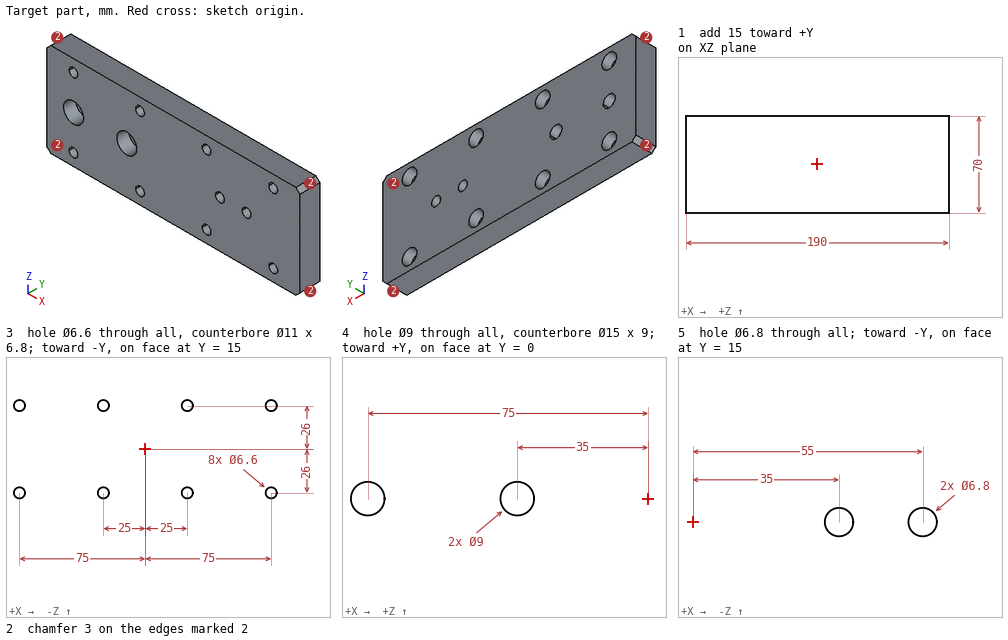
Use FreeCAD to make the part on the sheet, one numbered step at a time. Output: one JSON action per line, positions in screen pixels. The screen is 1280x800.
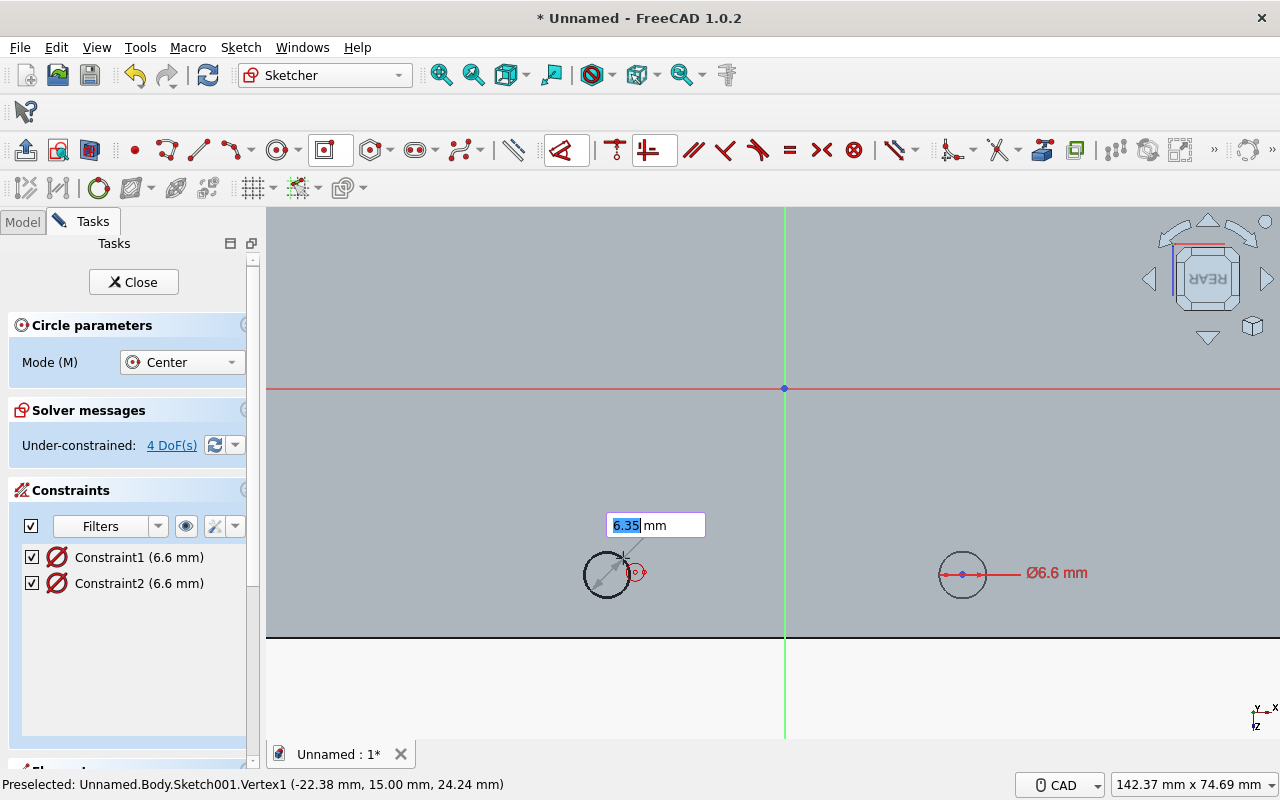
{"action": "type", "text": "6.6"}
{"action": "key", "text": "Return"}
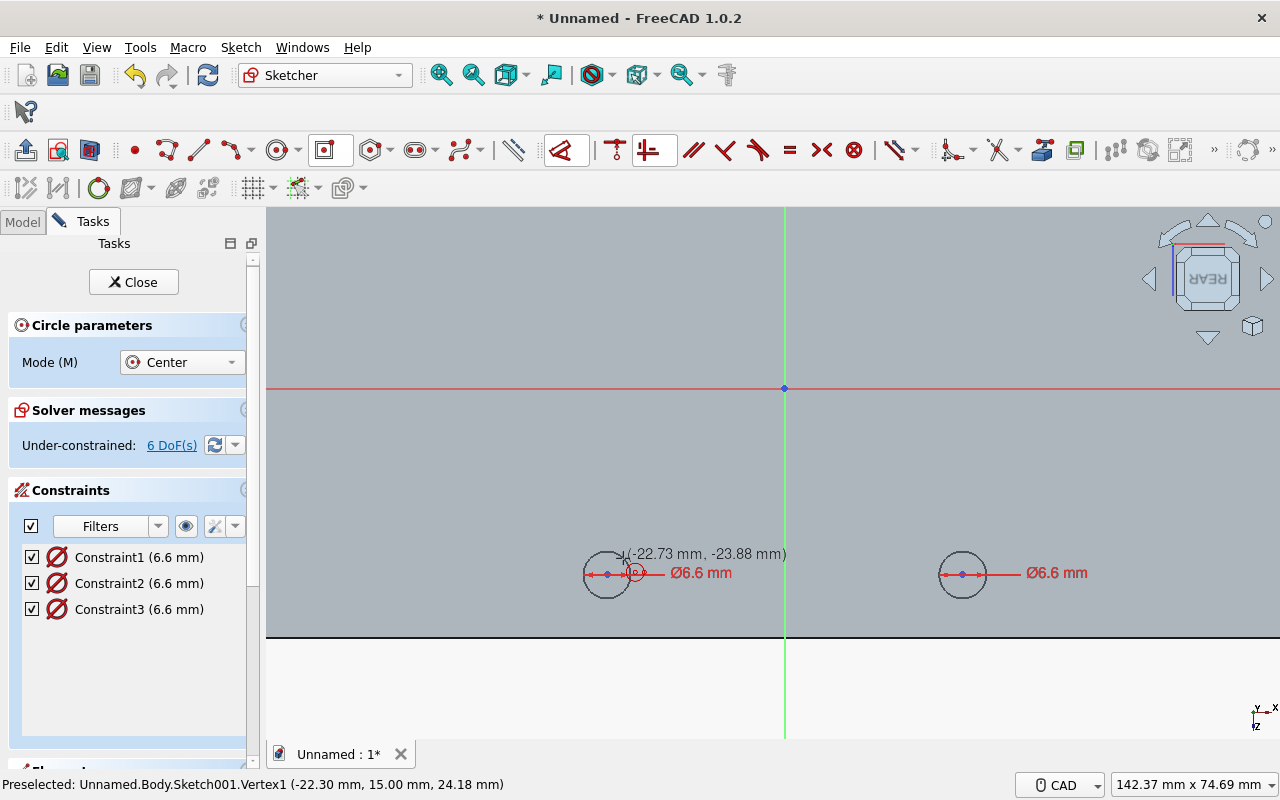
{"action": "scroll", "coordinate": [607, 575], "scroll_direction": "down", "scroll_amount": 3}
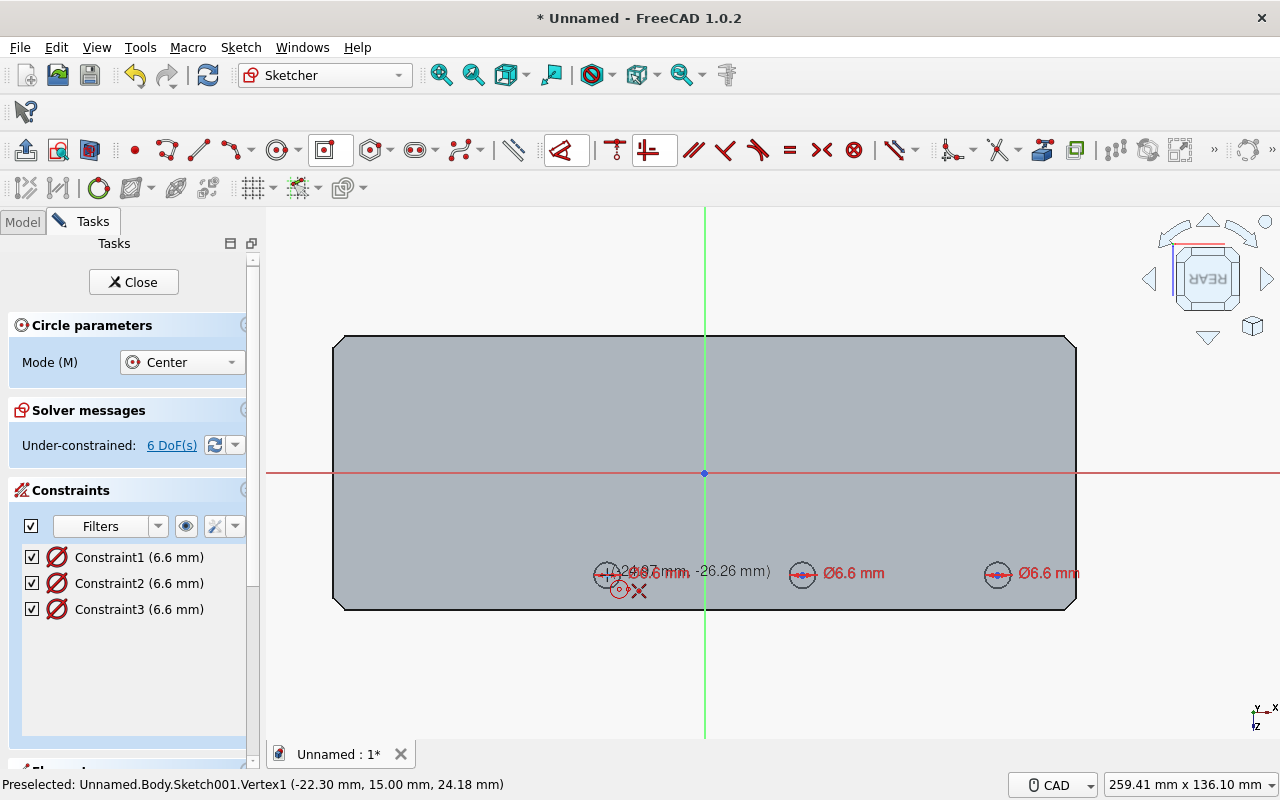
{"action": "scroll", "coordinate": [412, 575], "scroll_direction": "up", "scroll_amount": 3}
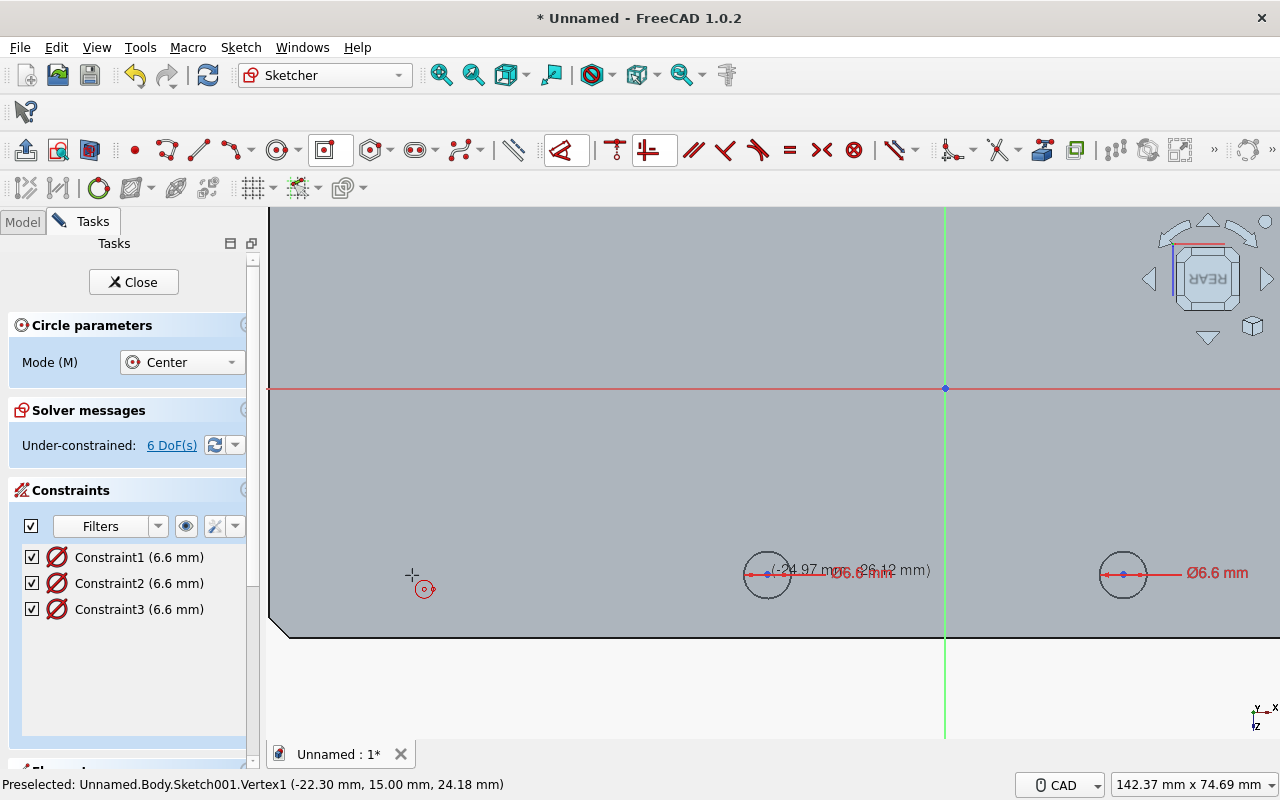
{"action": "left_click", "coordinate": [411, 574]}
{"action": "mouse_move", "coordinate": [428, 558]}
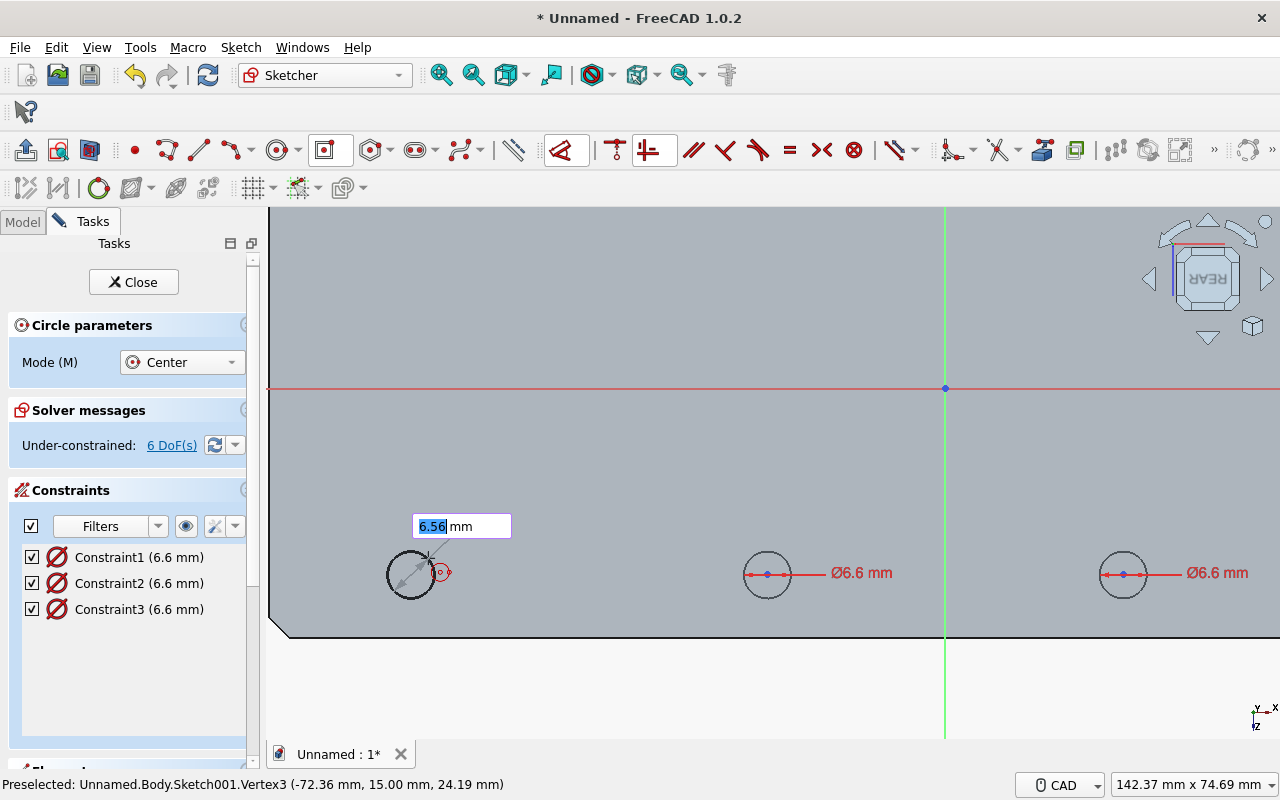
{"action": "type", "text": "6.6"}
{"action": "key", "text": "Return"}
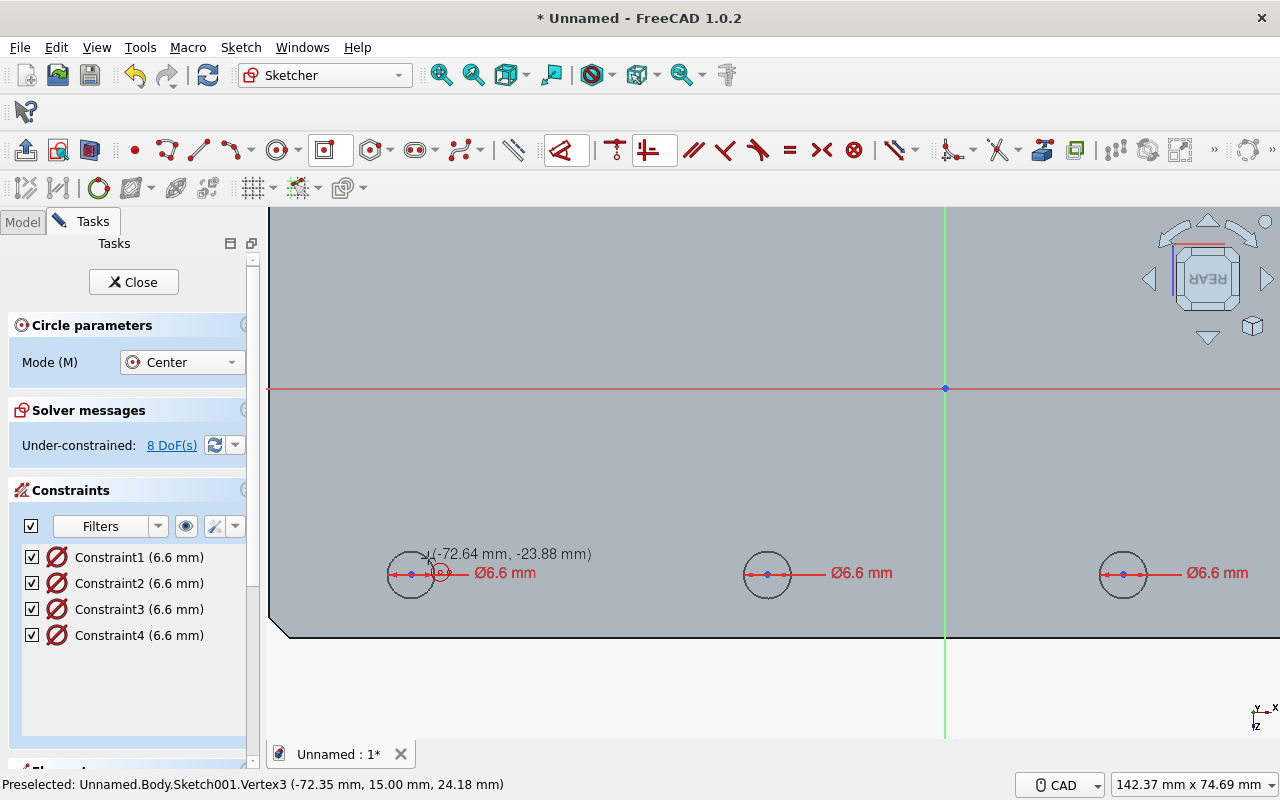
{"action": "scroll", "coordinate": [412, 575], "scroll_direction": "down", "scroll_amount": 3}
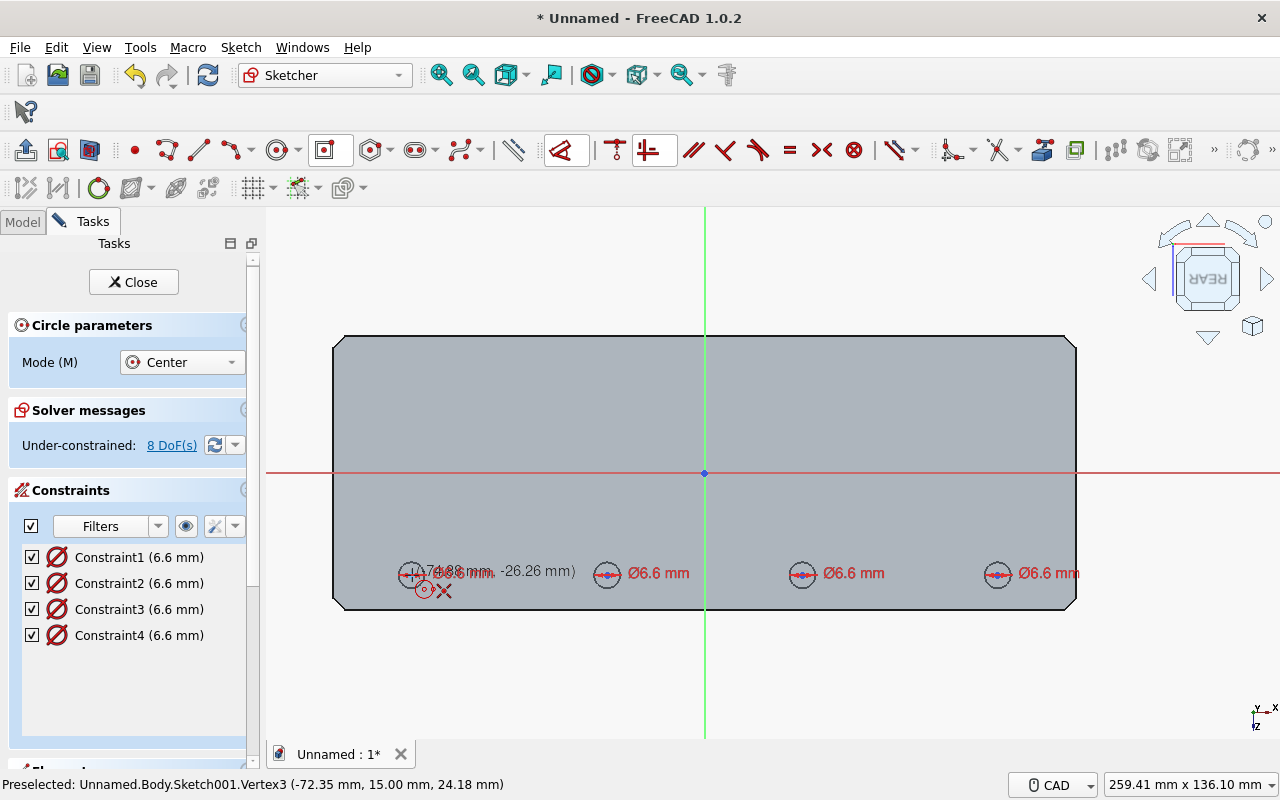
{"action": "scroll", "coordinate": [802, 372], "scroll_direction": "up", "scroll_amount": 3}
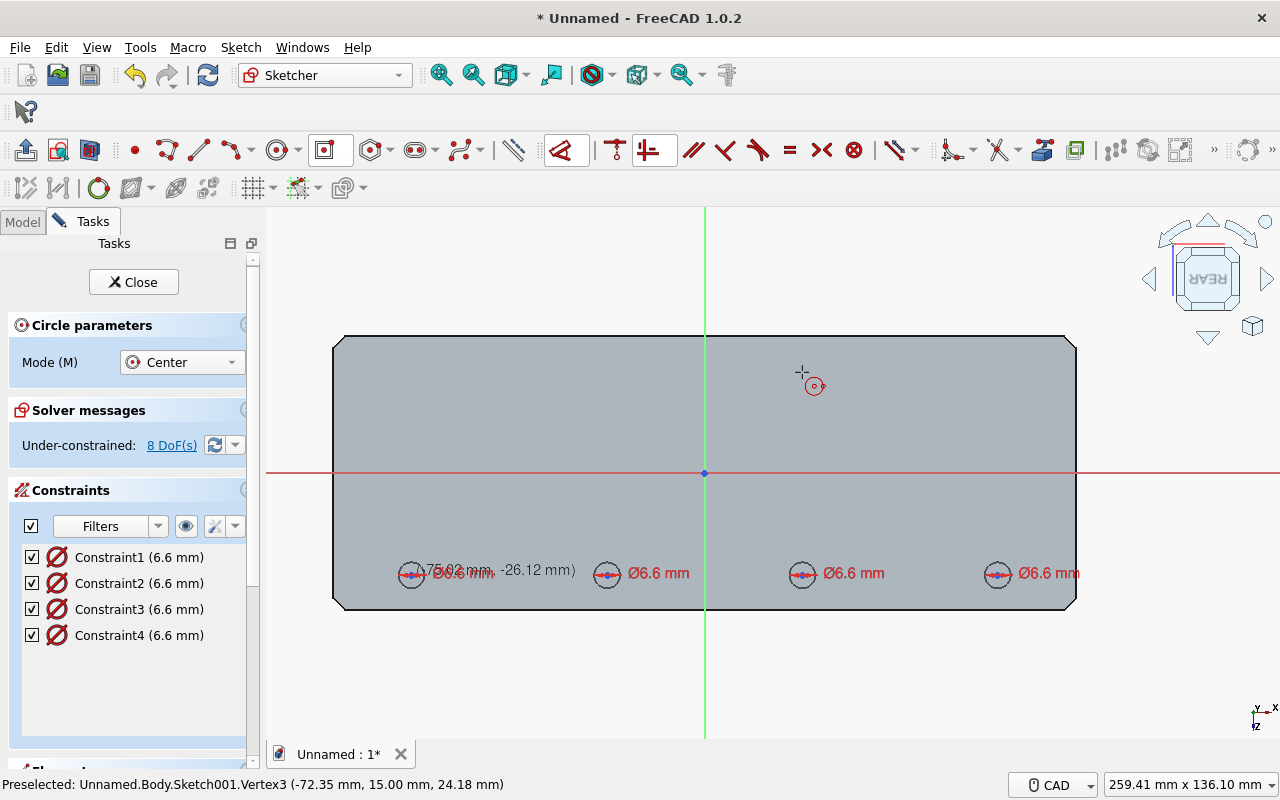
{"action": "left_click", "coordinate": [802, 371]}
{"action": "mouse_move", "coordinate": [819, 354]}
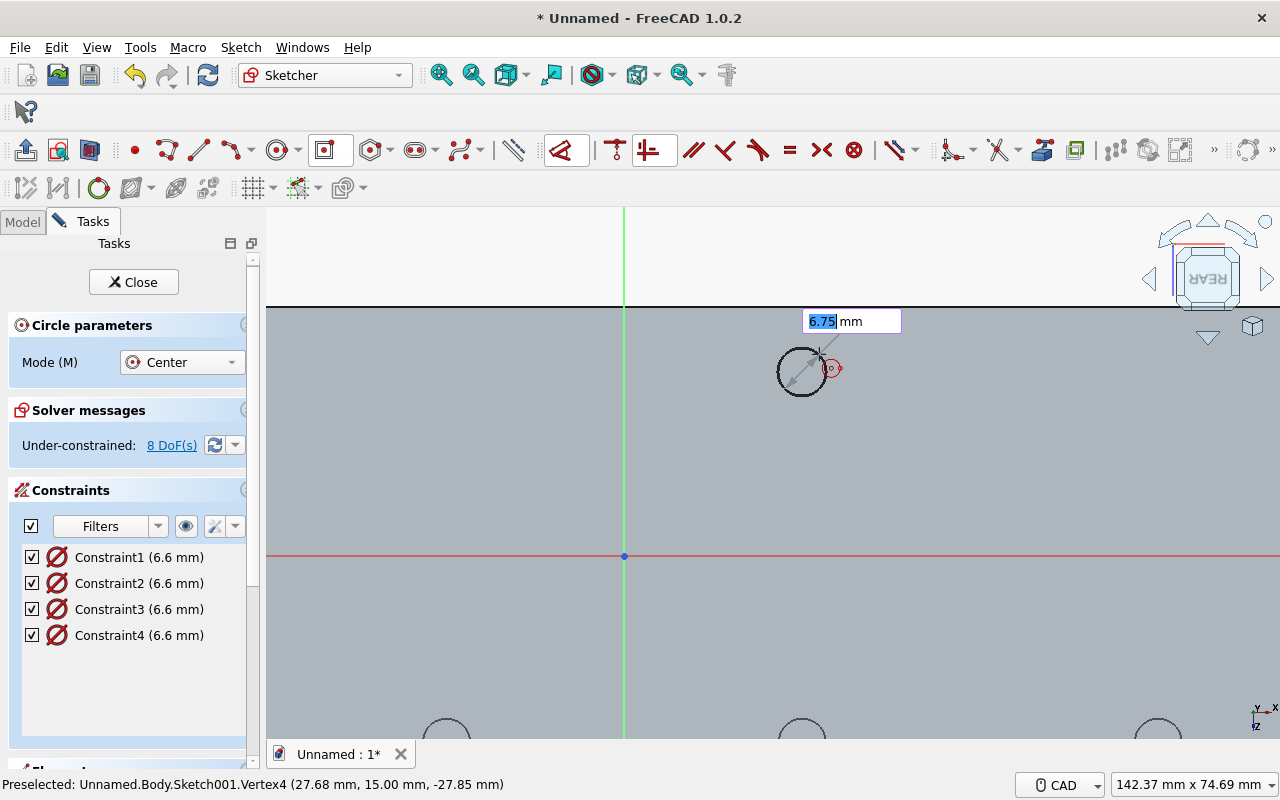
{"action": "type", "text": "6.6"}
{"action": "key", "text": "Return"}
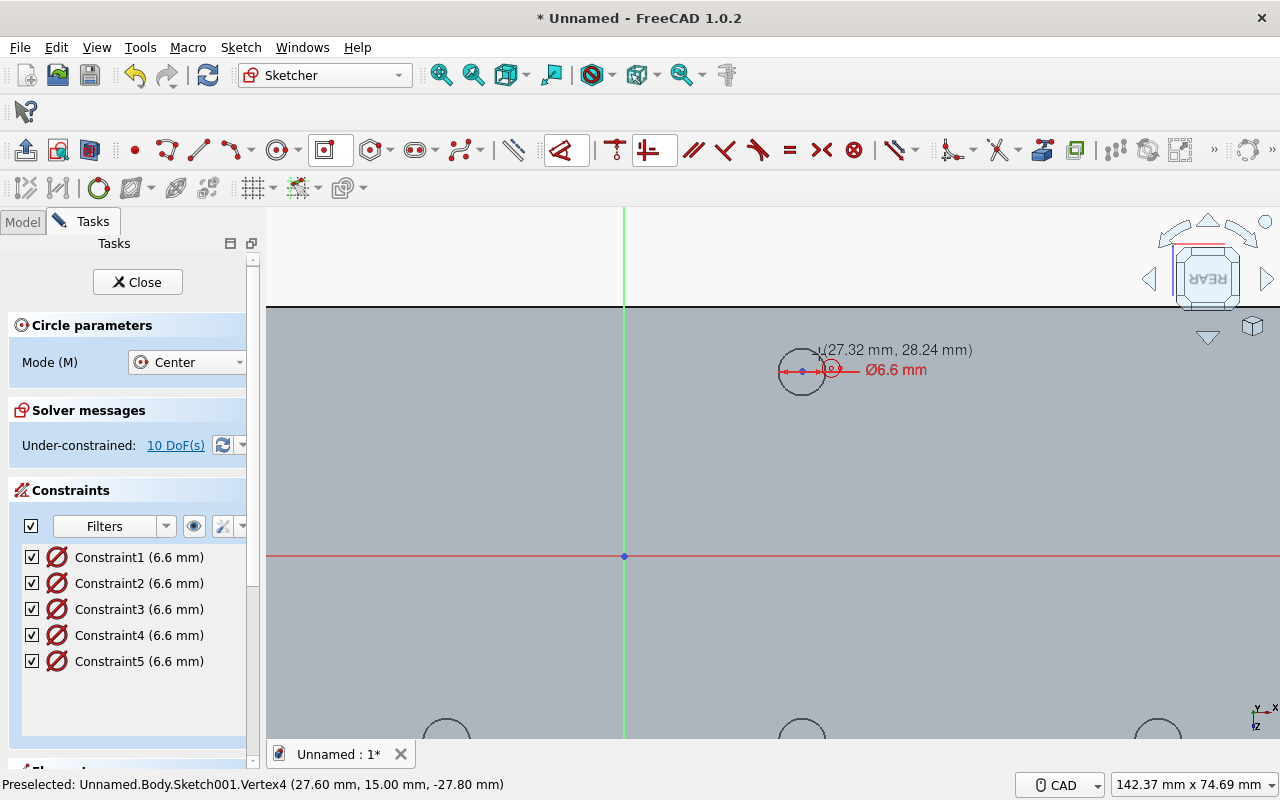
{"action": "left_click", "coordinate": [446, 371]}
{"action": "mouse_move", "coordinate": [463, 354]}